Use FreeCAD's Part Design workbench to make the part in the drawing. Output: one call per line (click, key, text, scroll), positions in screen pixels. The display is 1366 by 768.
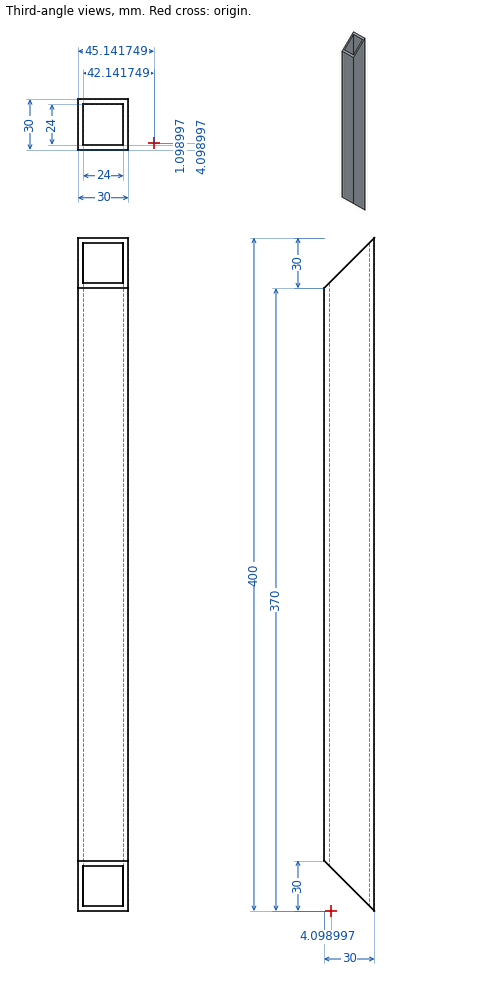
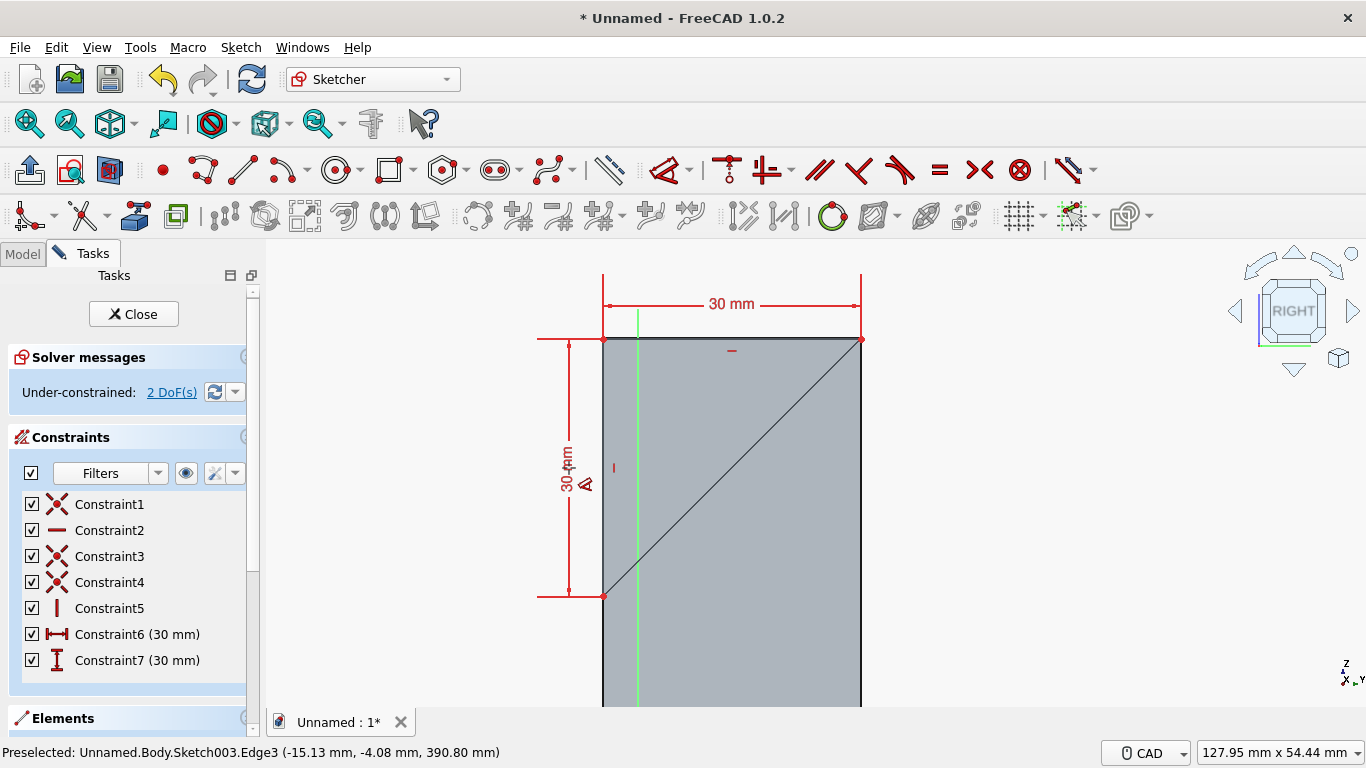
click(603, 597)
click(569, 638)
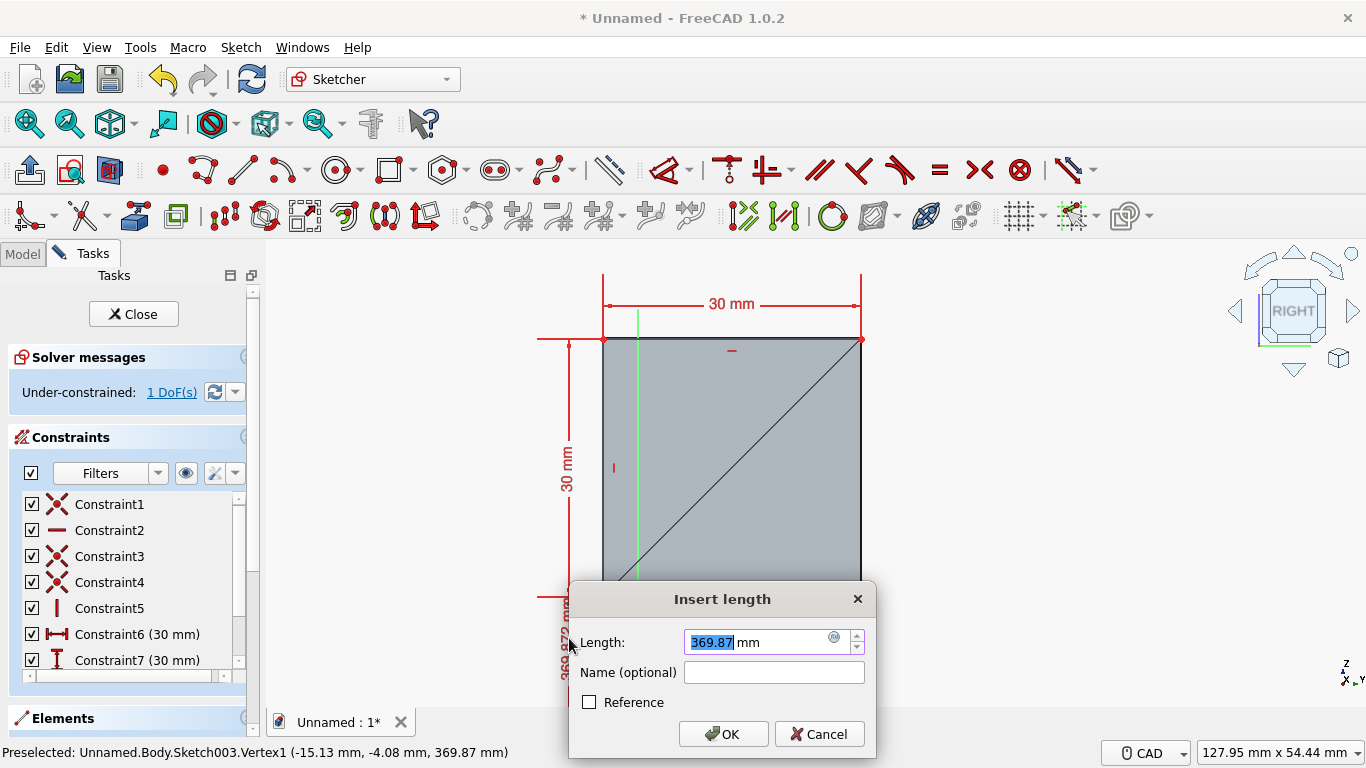
text(370)
key(Return)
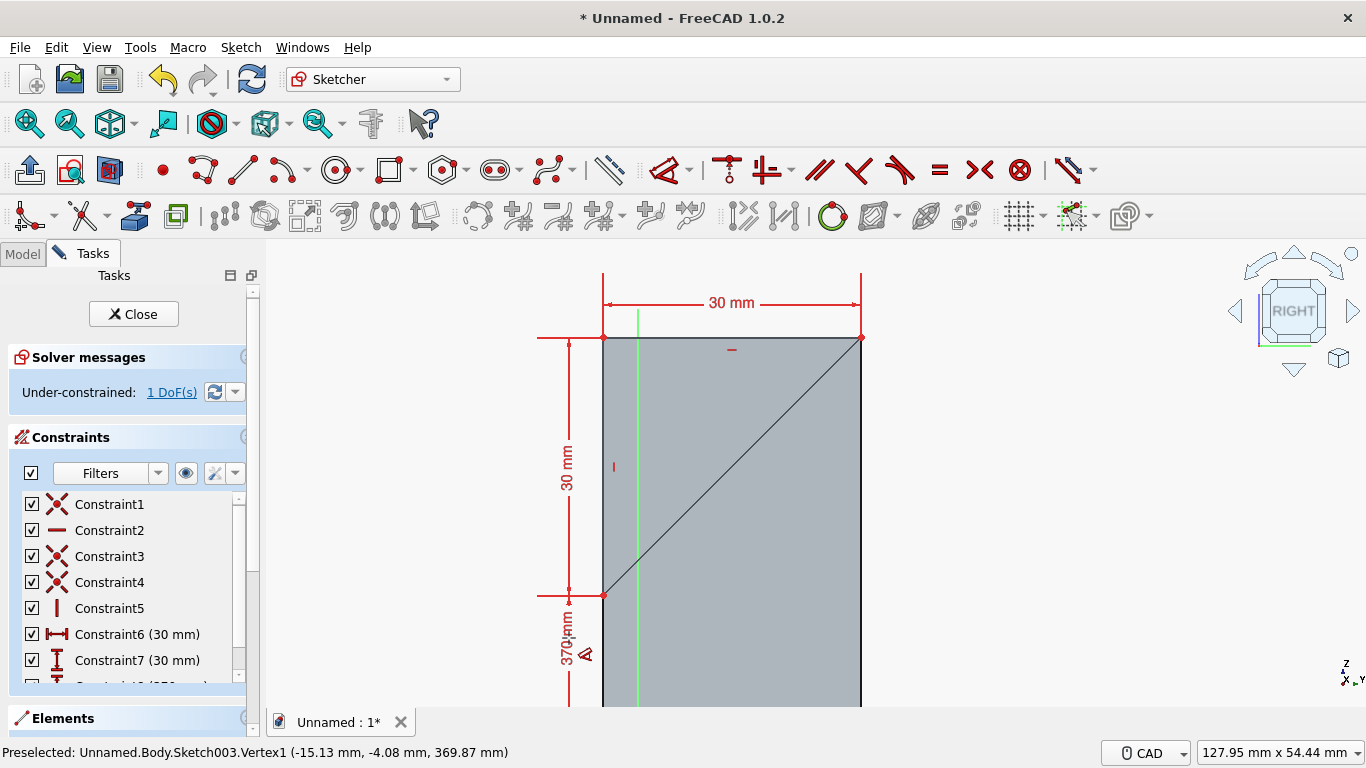
click(603, 596)
click(621, 538)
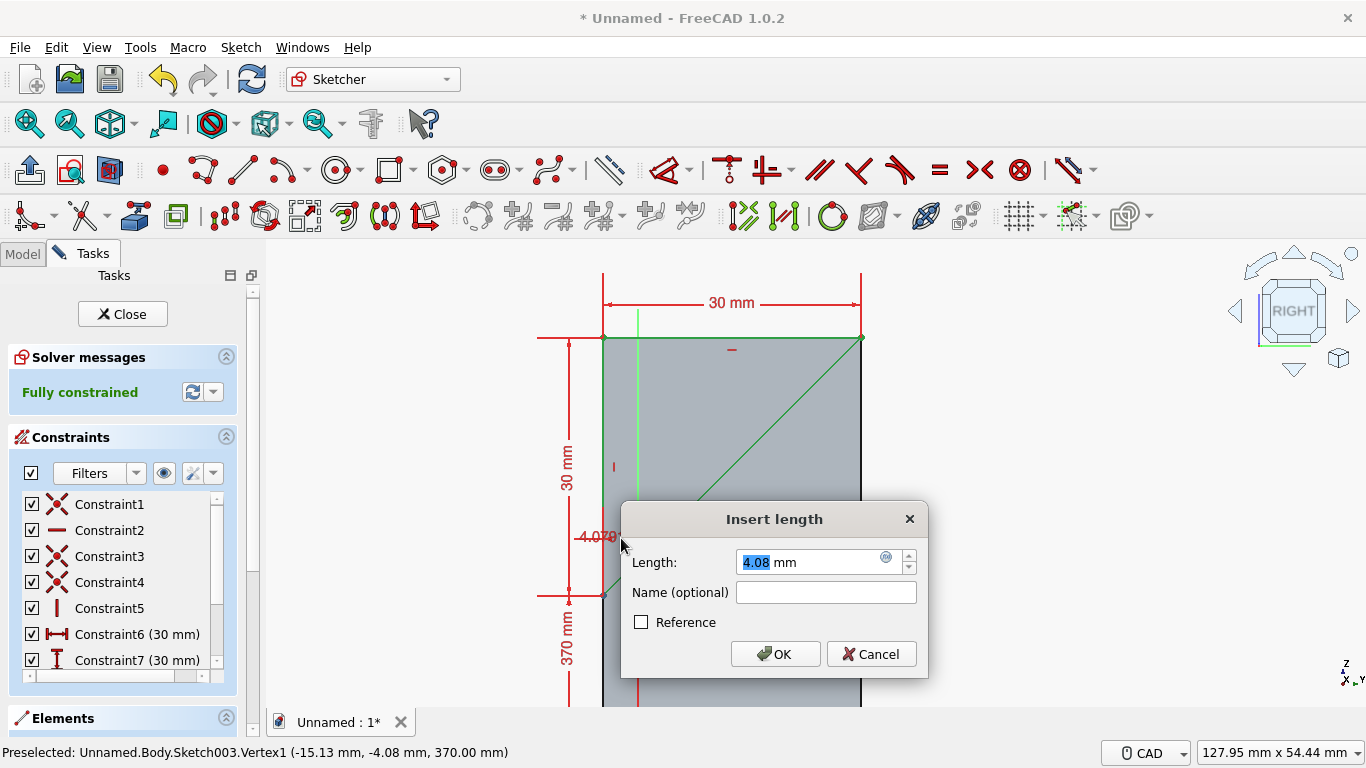
text(4.098997)
key(Return)
key(Escape)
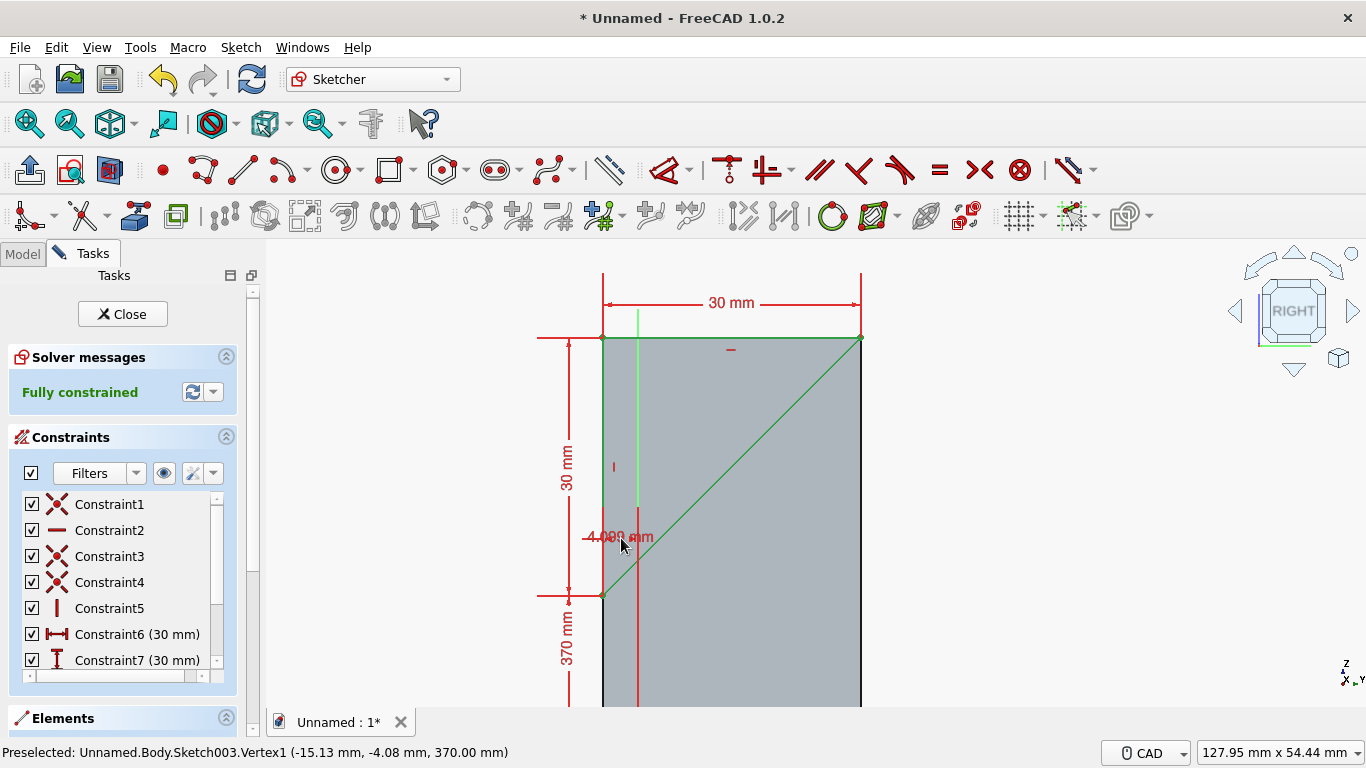
click(123, 314)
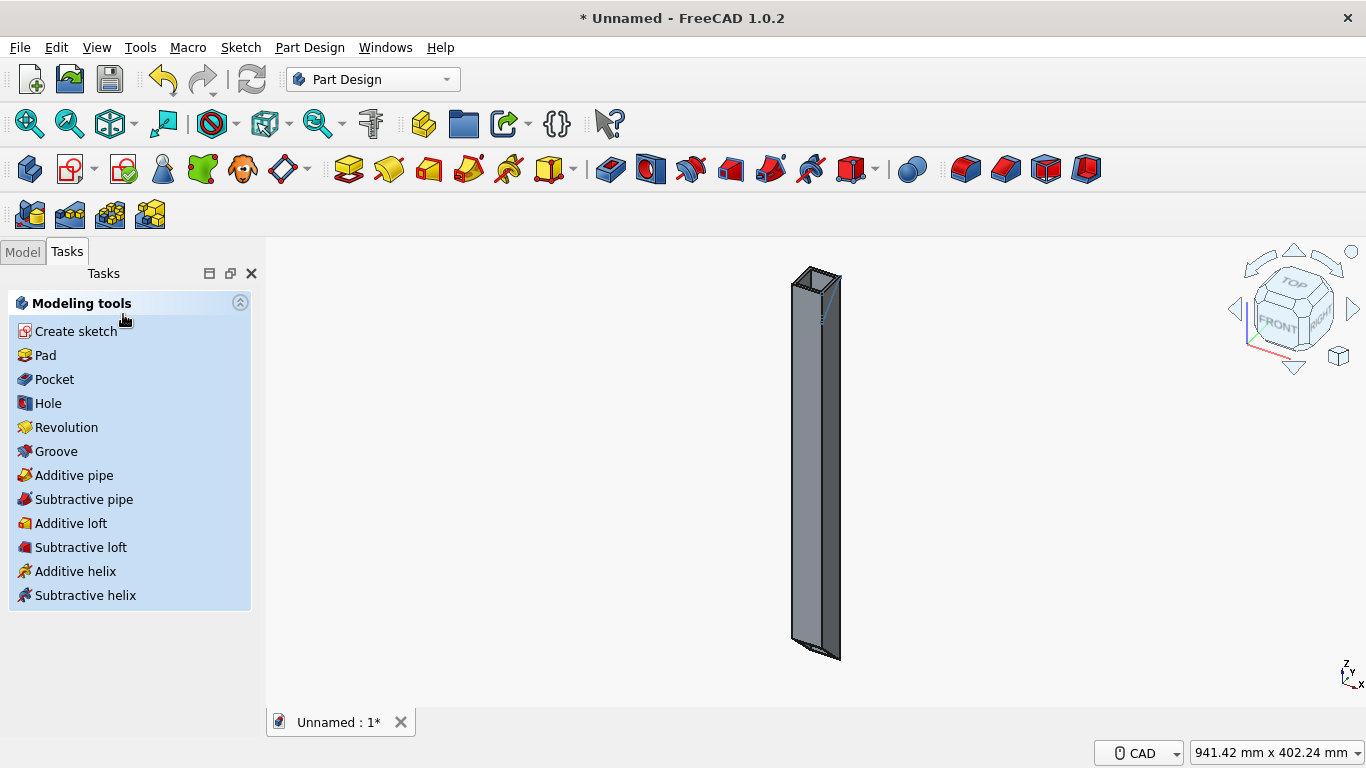
click(612, 170)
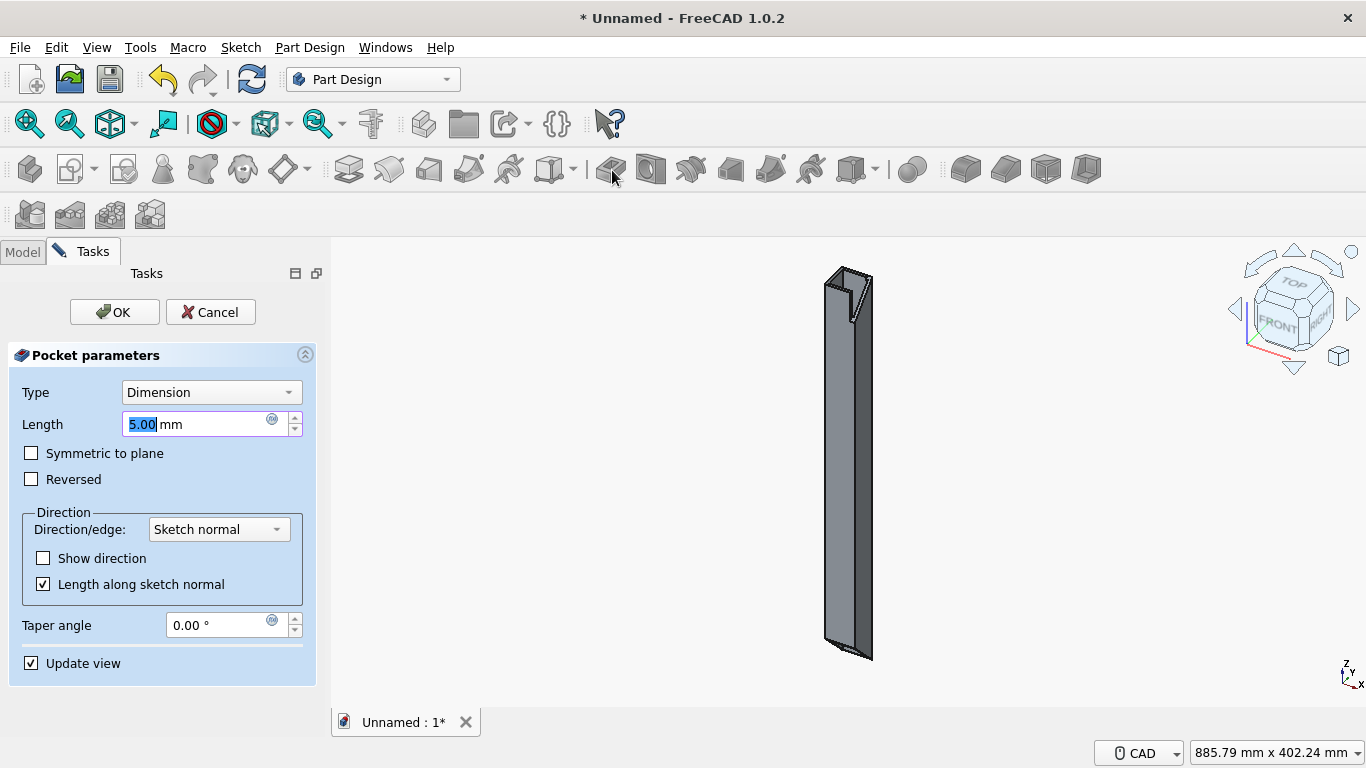
click(212, 392)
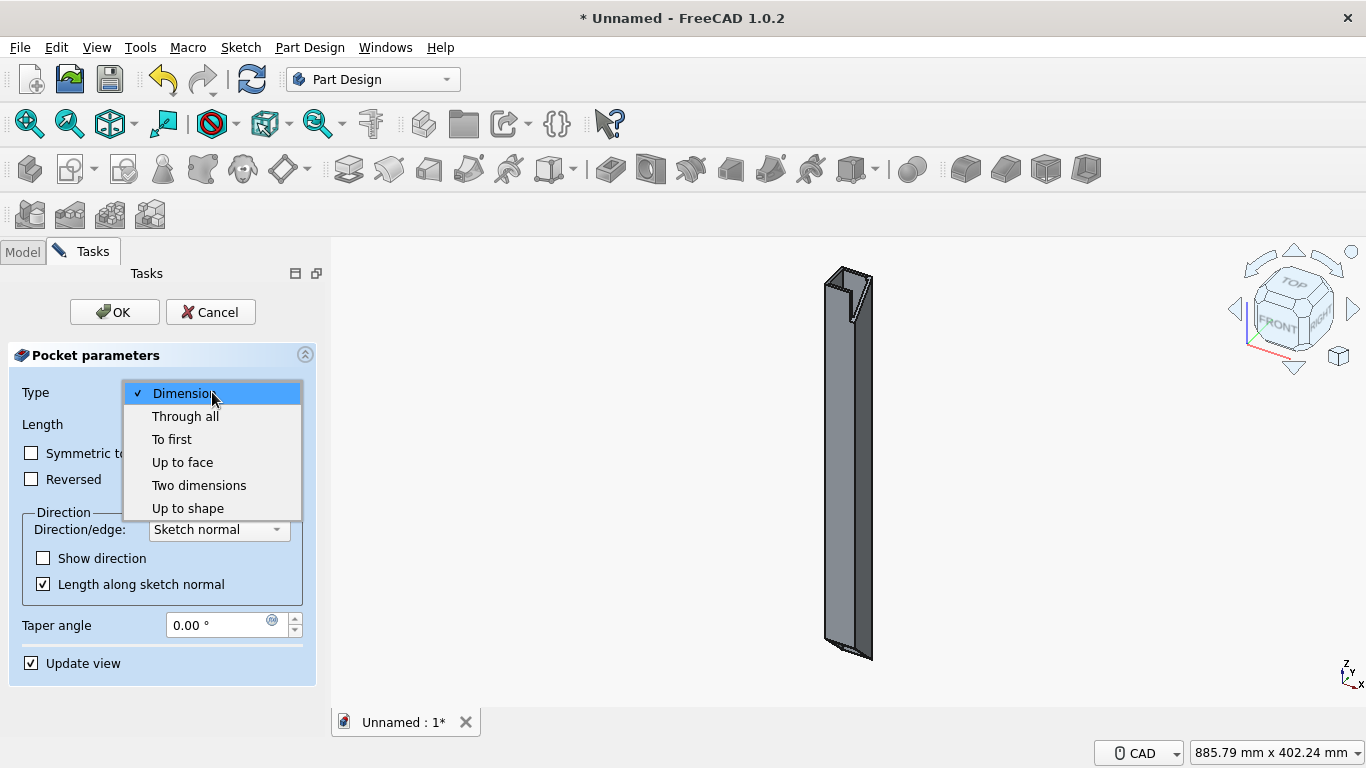
click(212, 416)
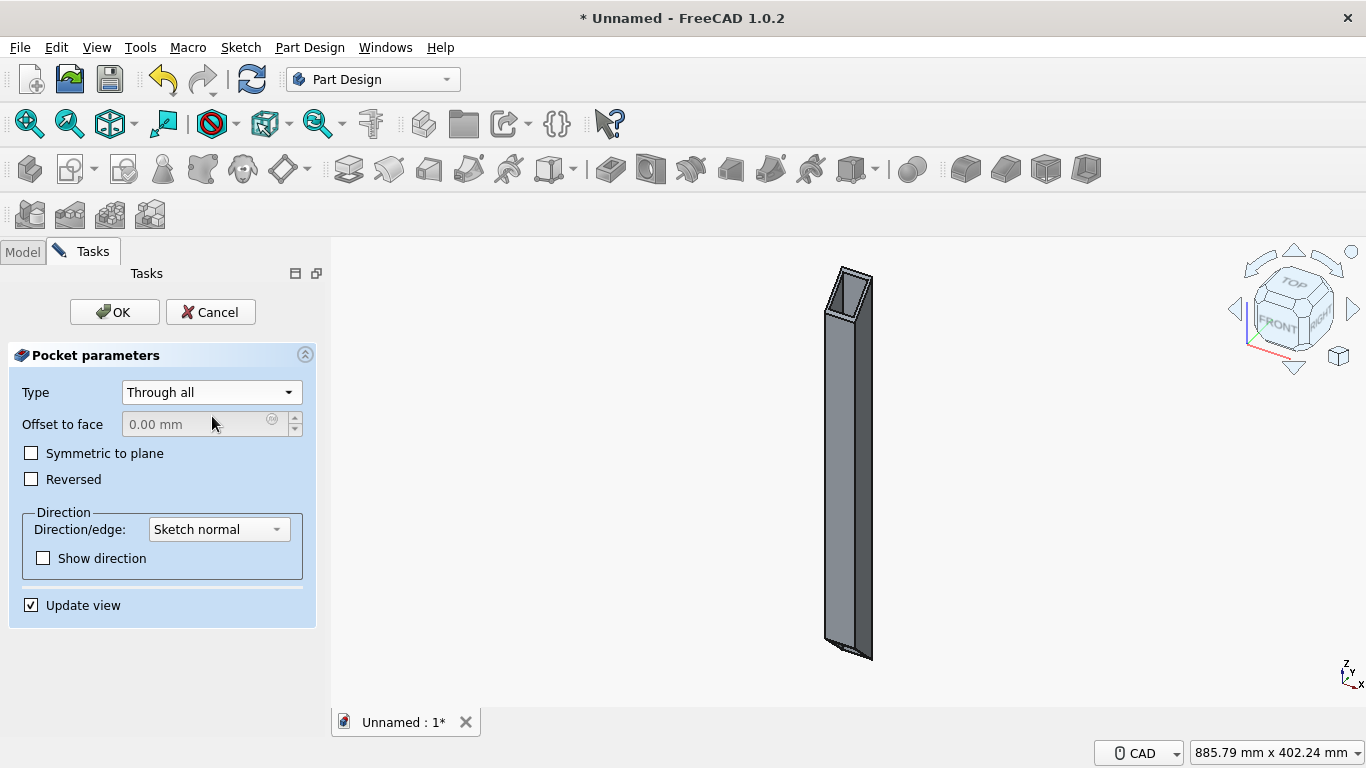
click(115, 312)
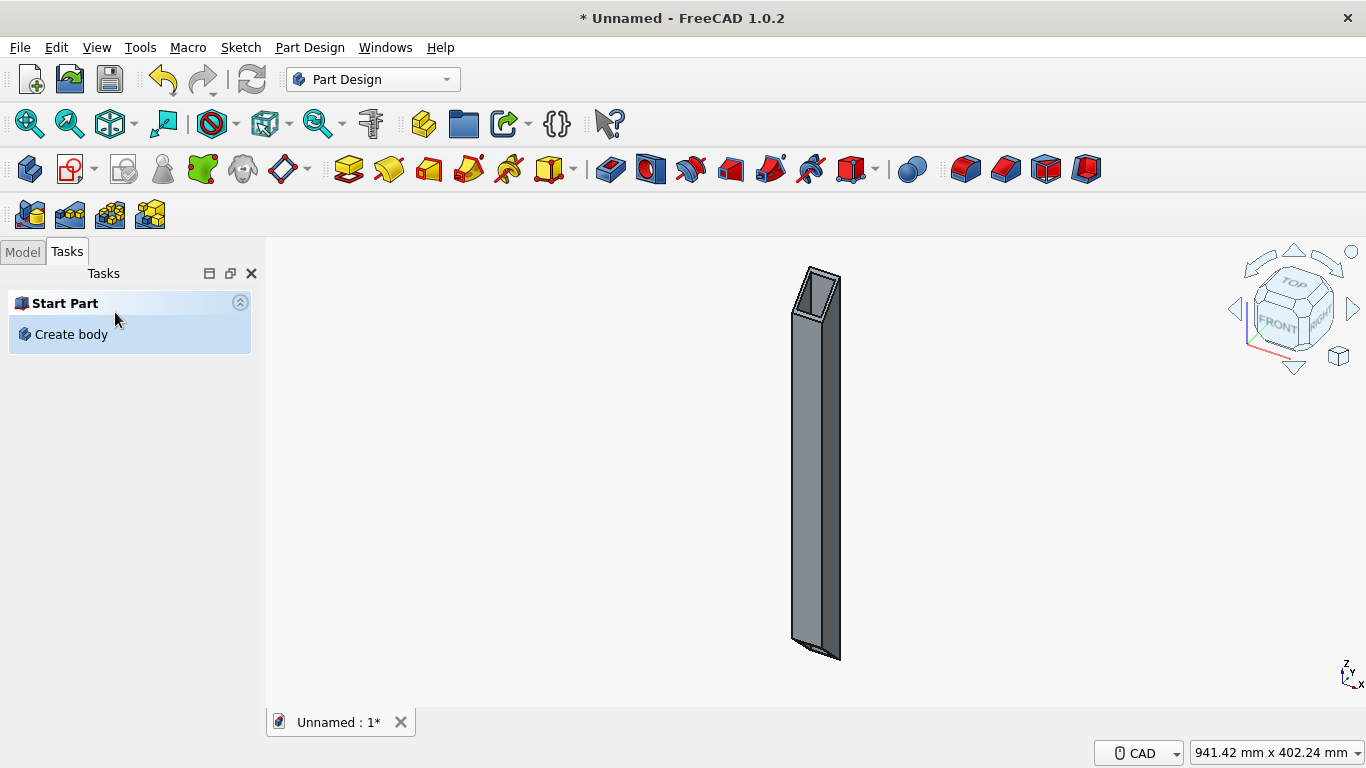
key(0)